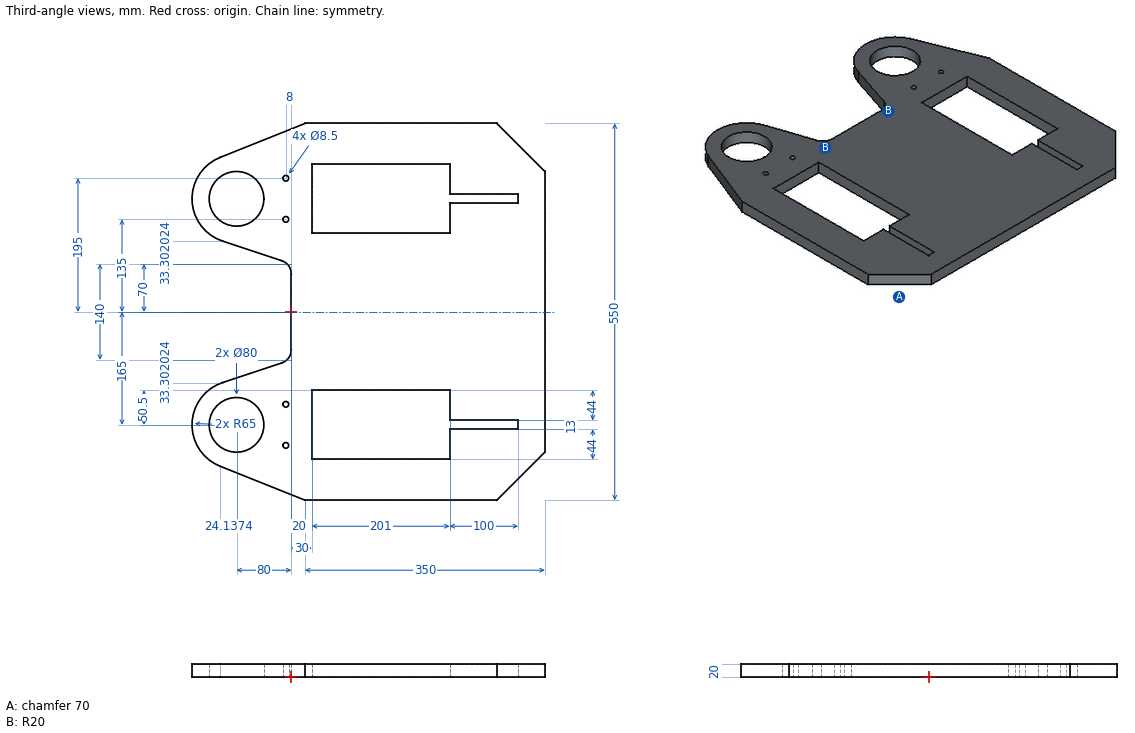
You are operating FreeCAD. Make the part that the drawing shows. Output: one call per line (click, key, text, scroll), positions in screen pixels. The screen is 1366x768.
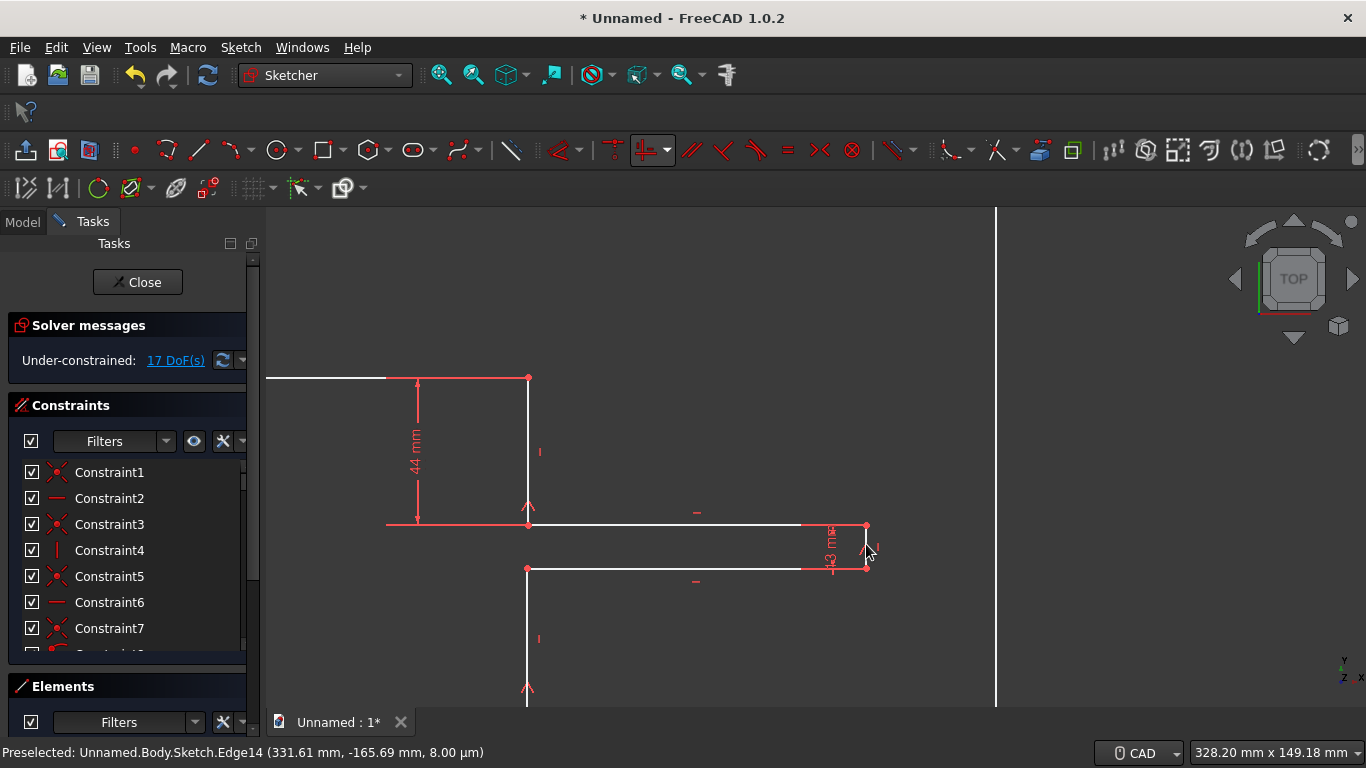
scroll(869, 550, down, 9)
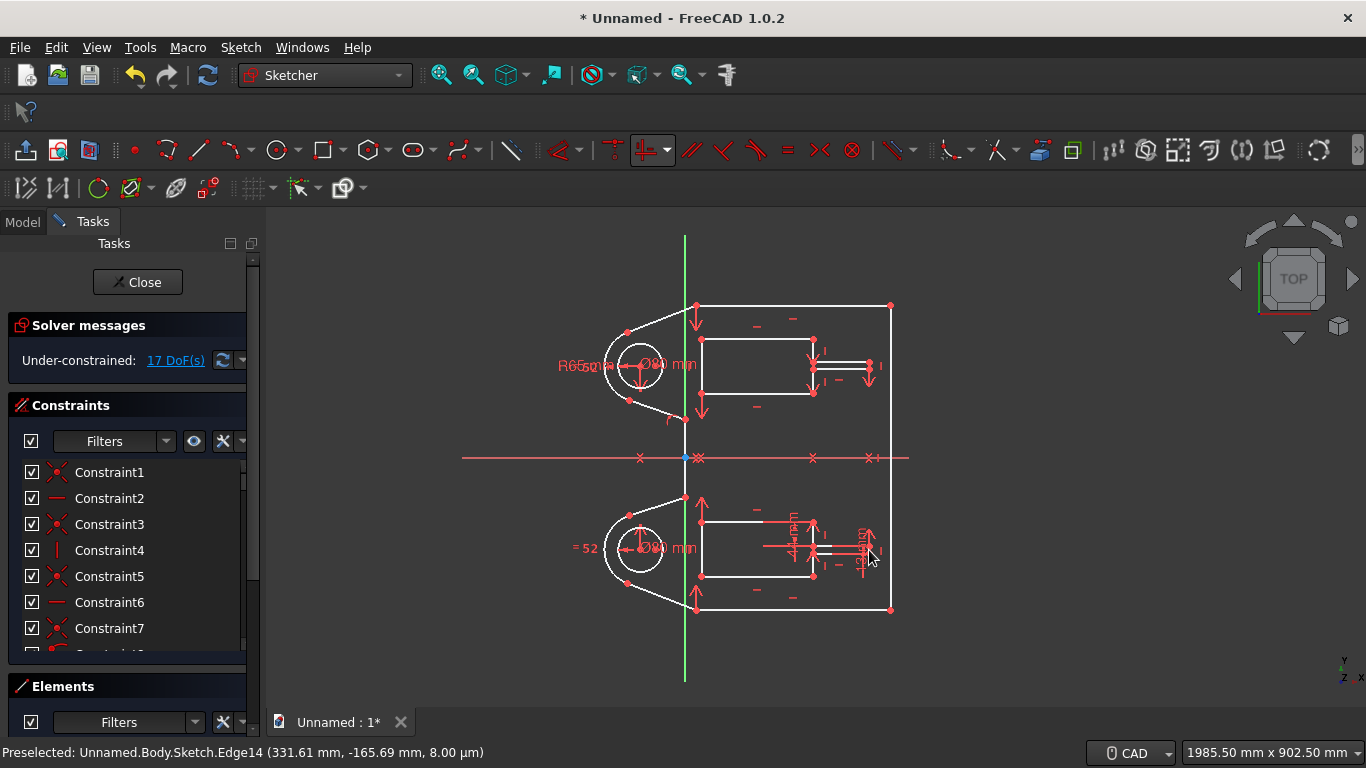
scroll(813, 561, up, 4)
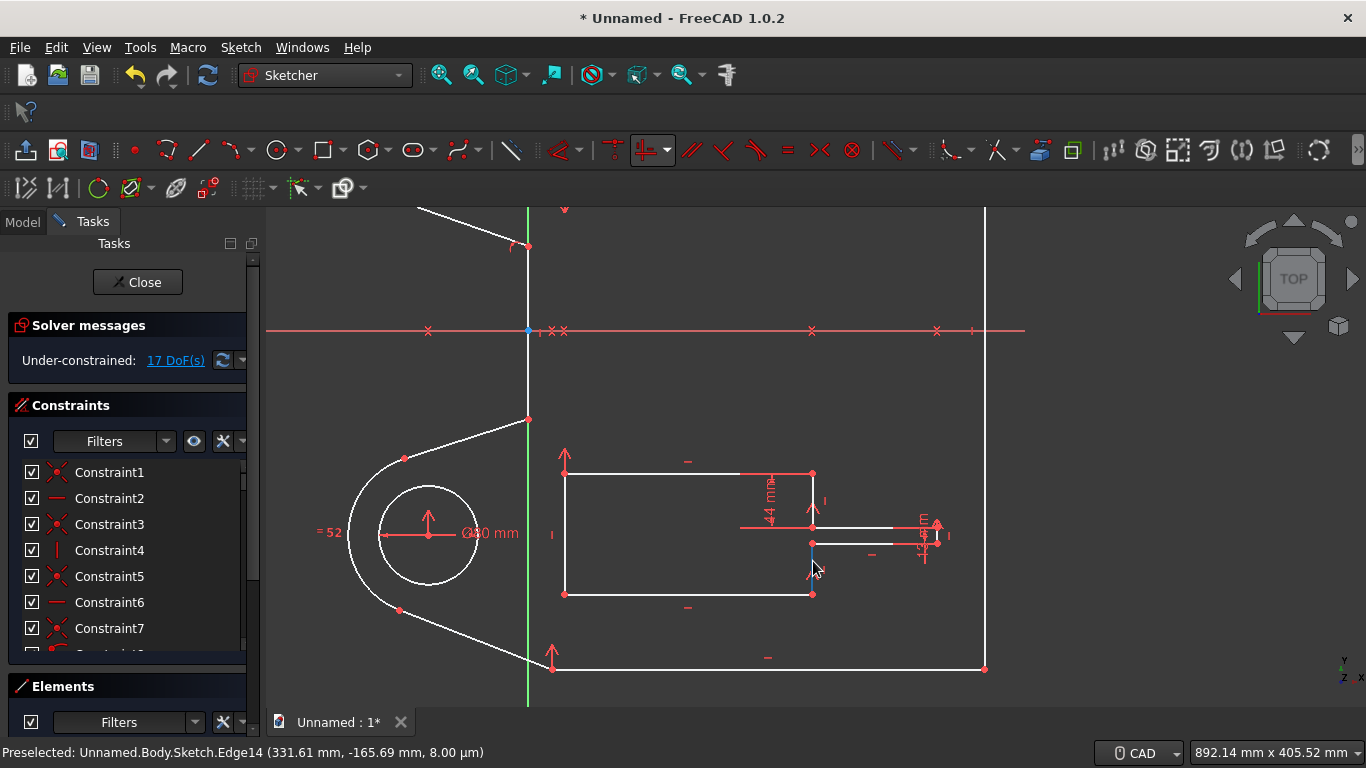
click(812, 559)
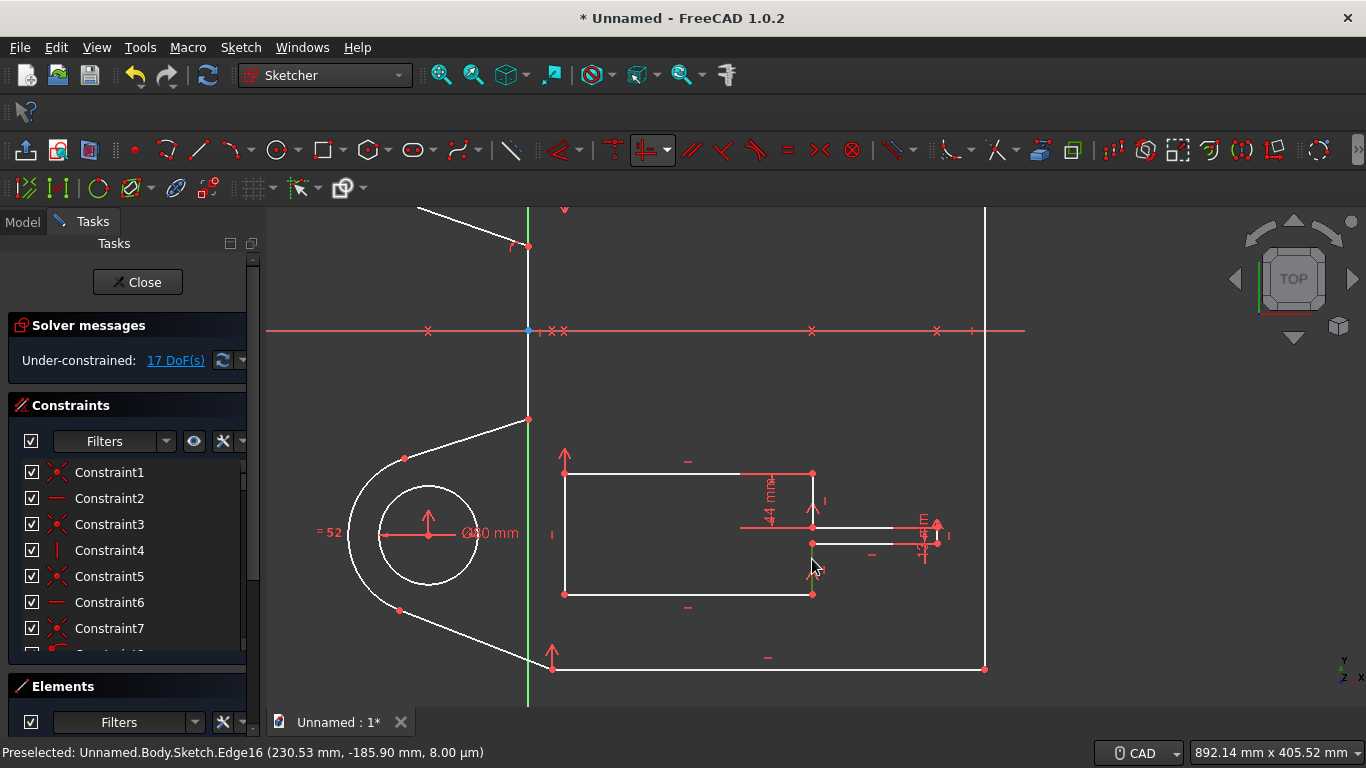
click(582, 150)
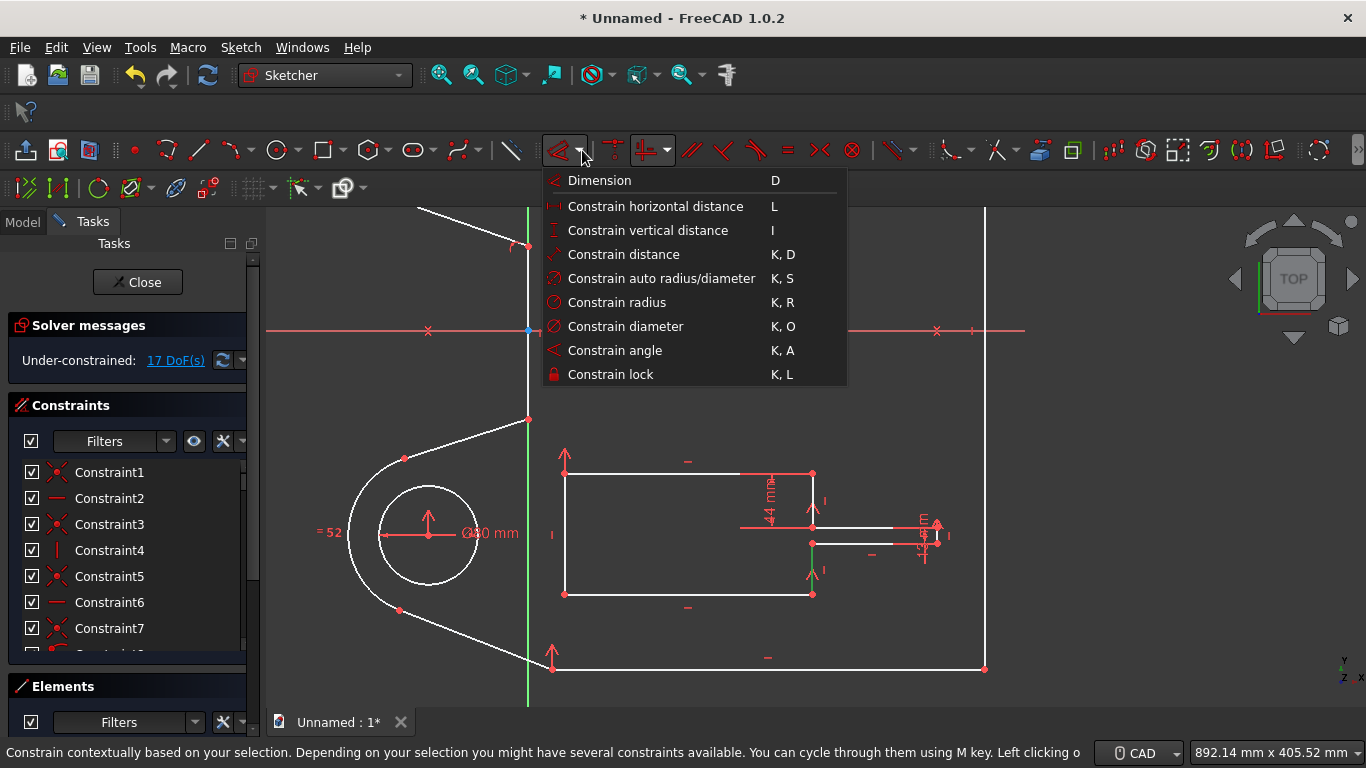
click(695, 230)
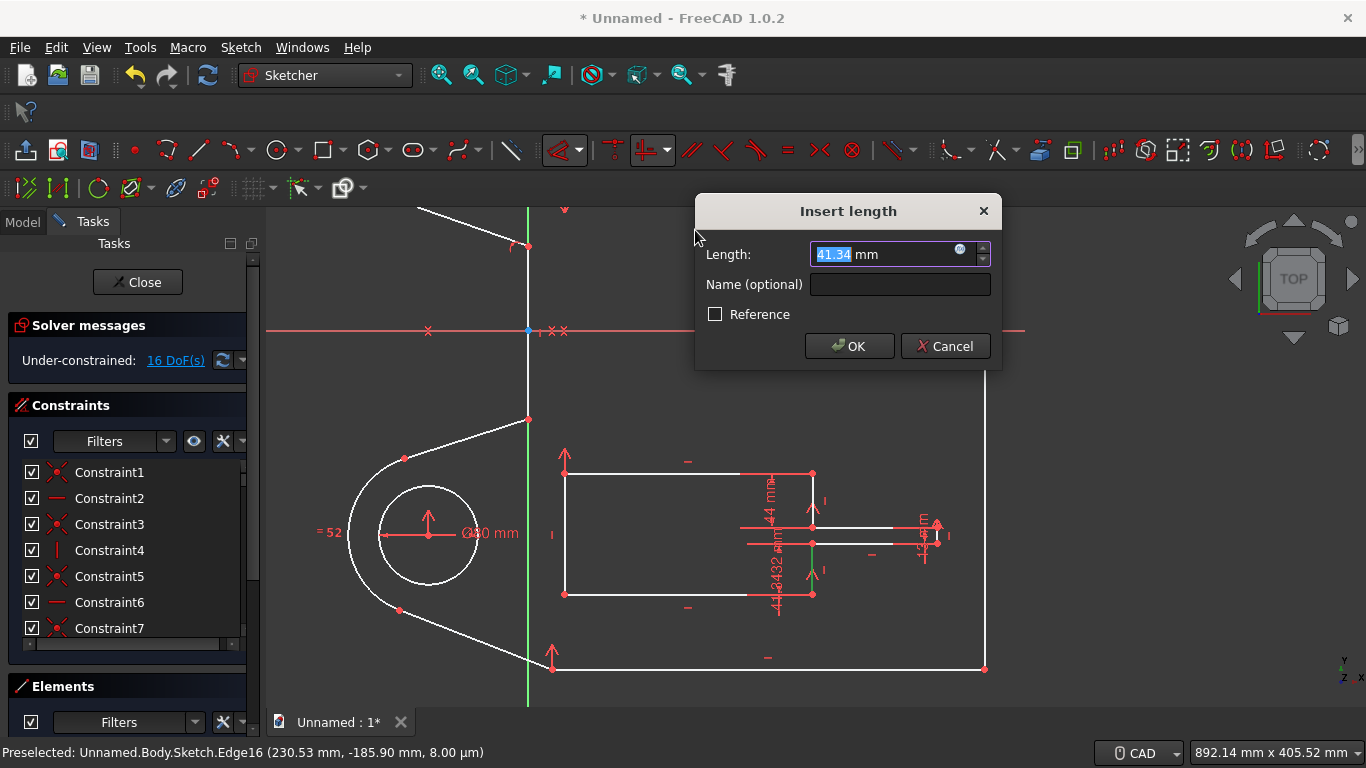
text(44)
key(Return)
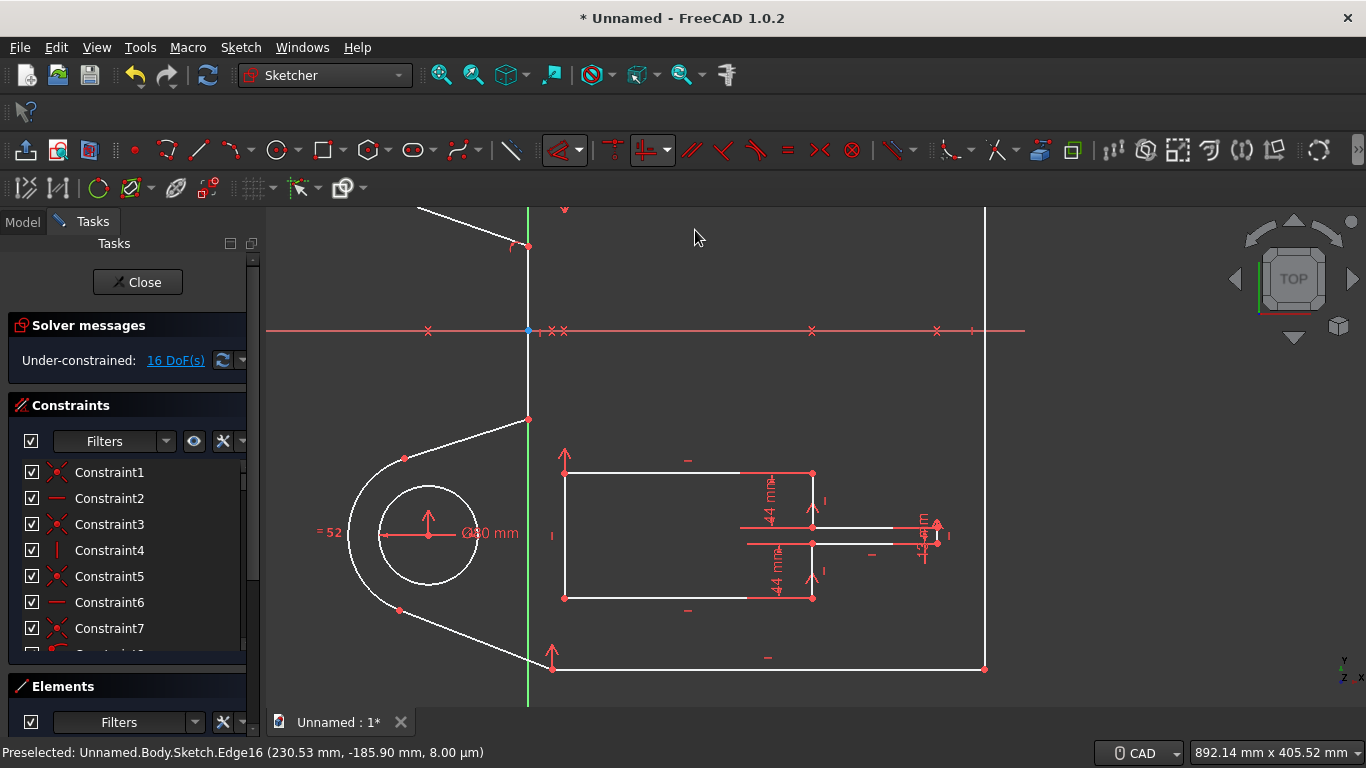
click(428, 535)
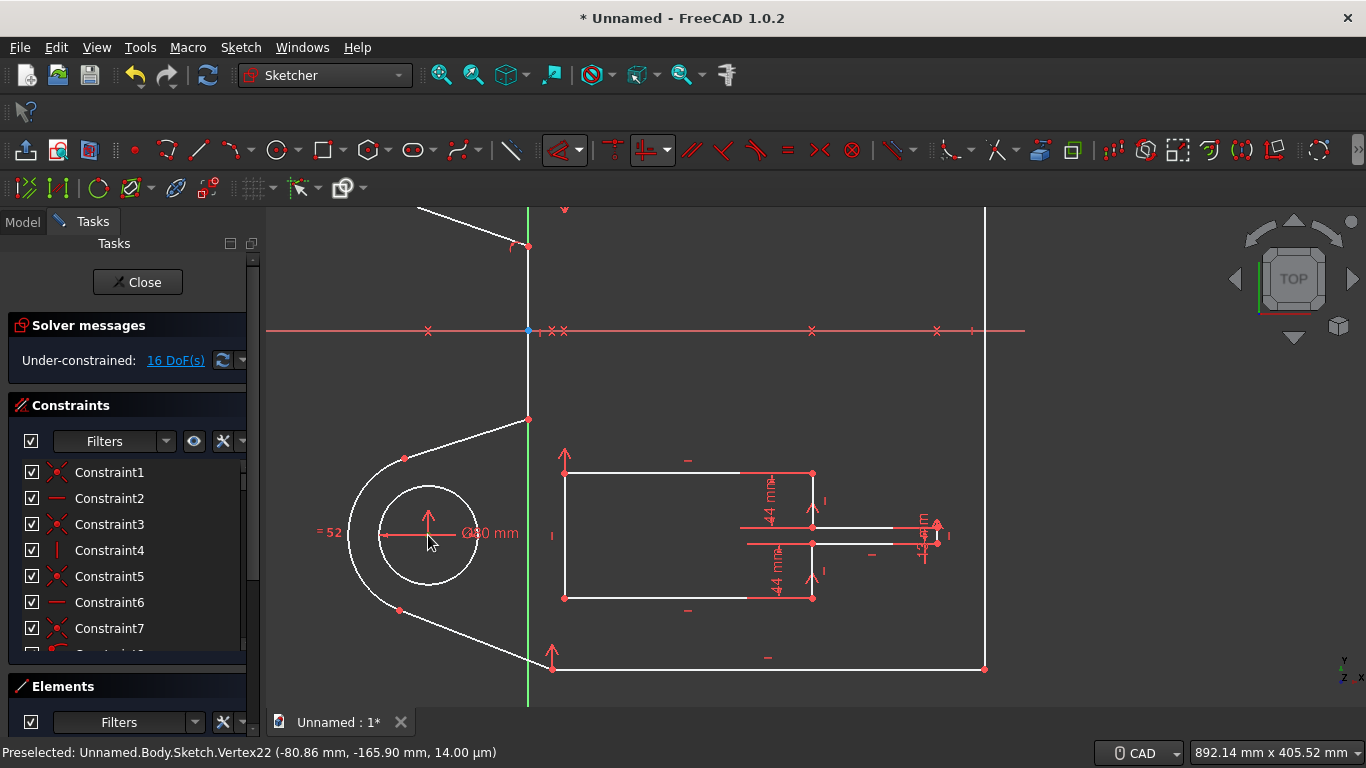
key(l)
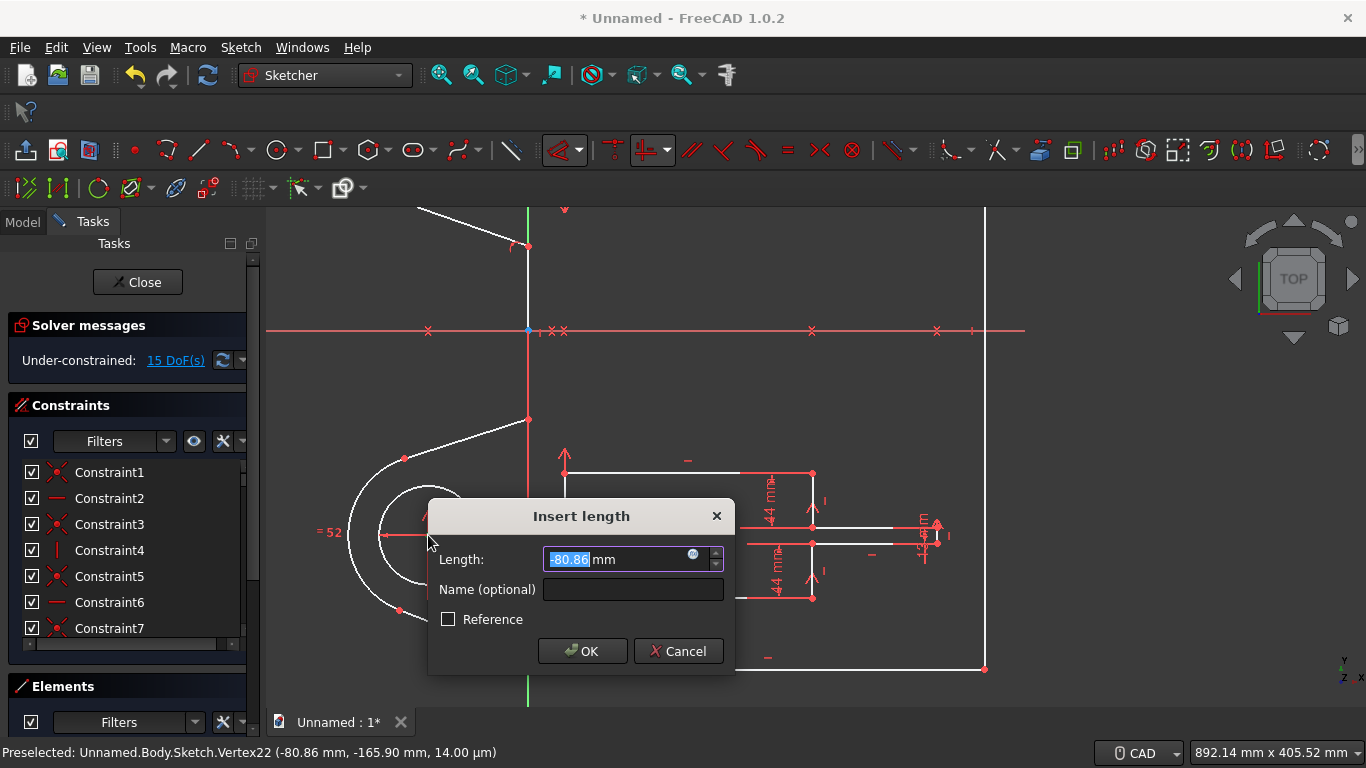
text(-80)
key(Return)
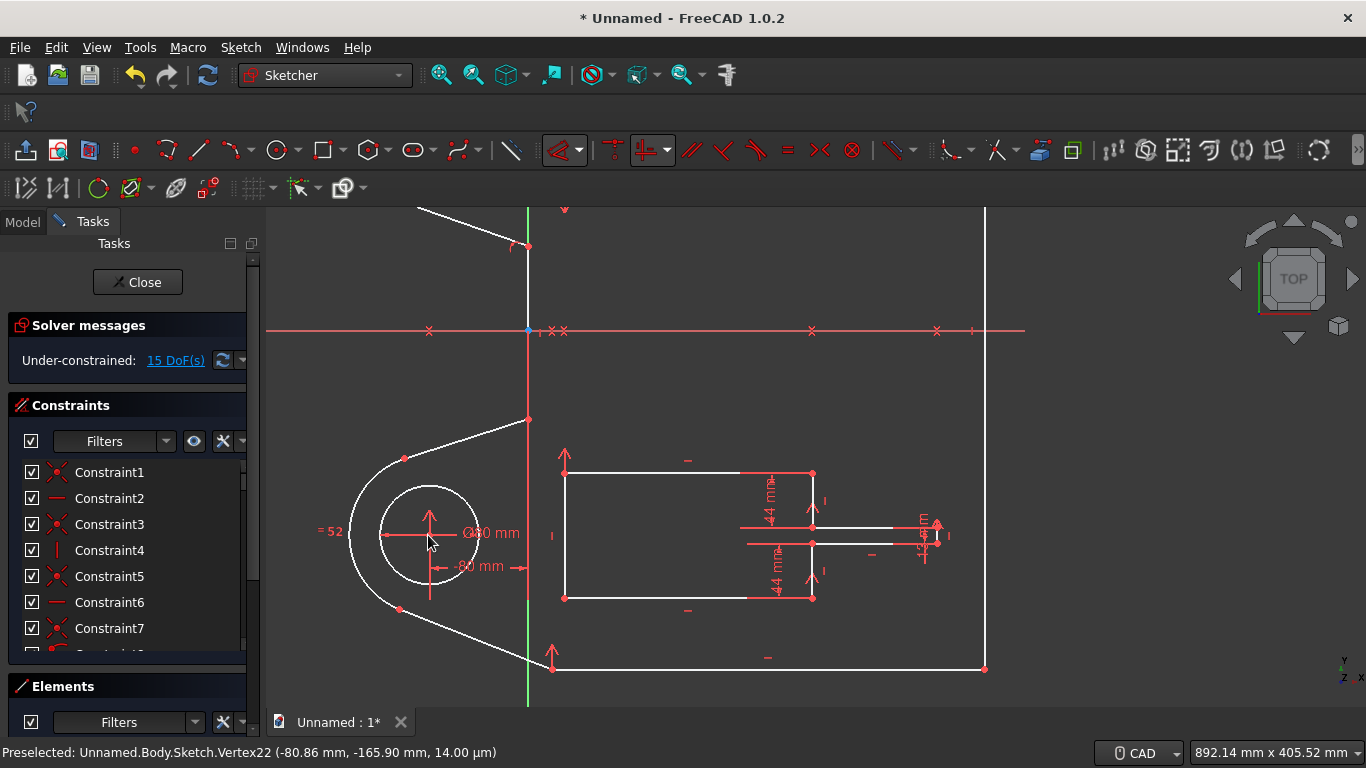
click(682, 670)